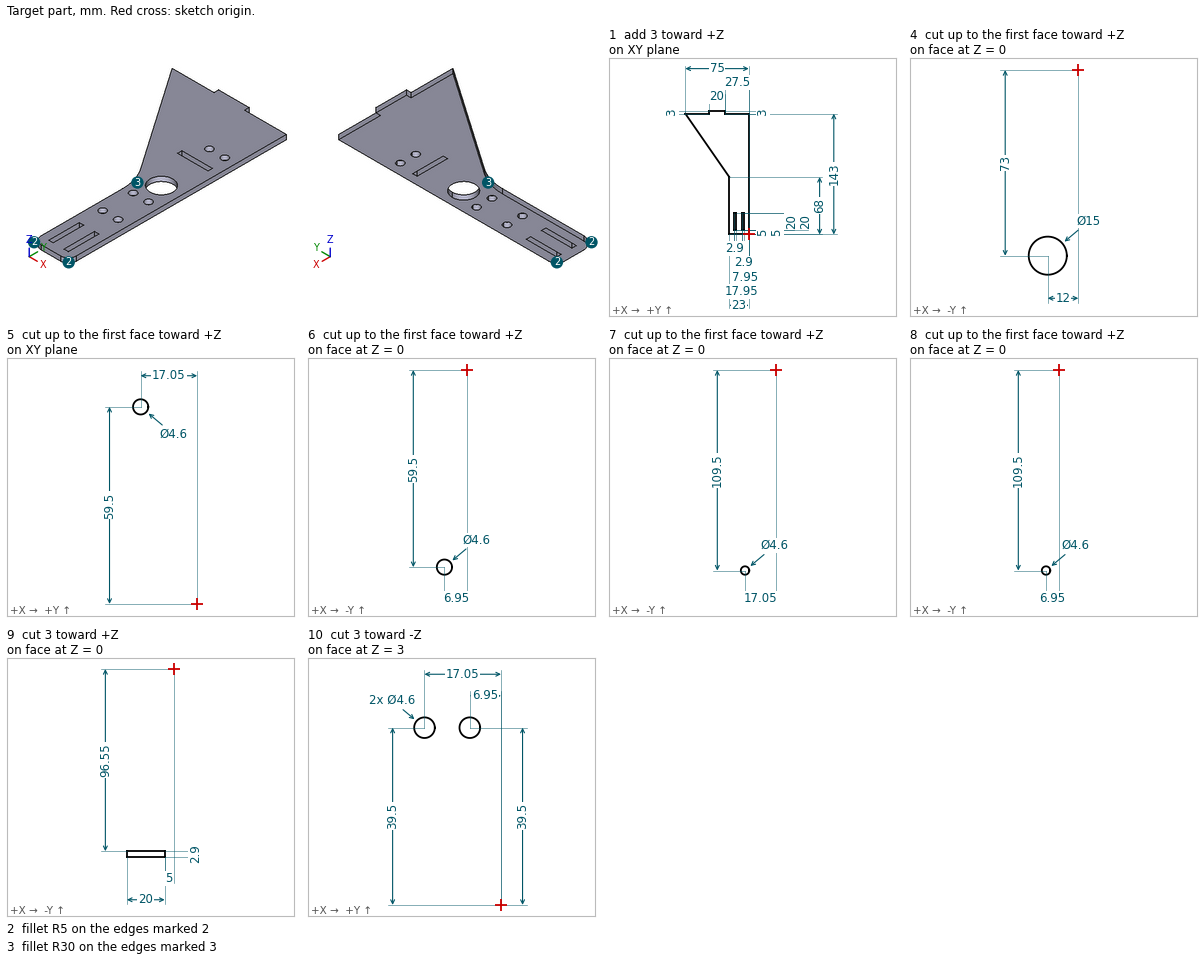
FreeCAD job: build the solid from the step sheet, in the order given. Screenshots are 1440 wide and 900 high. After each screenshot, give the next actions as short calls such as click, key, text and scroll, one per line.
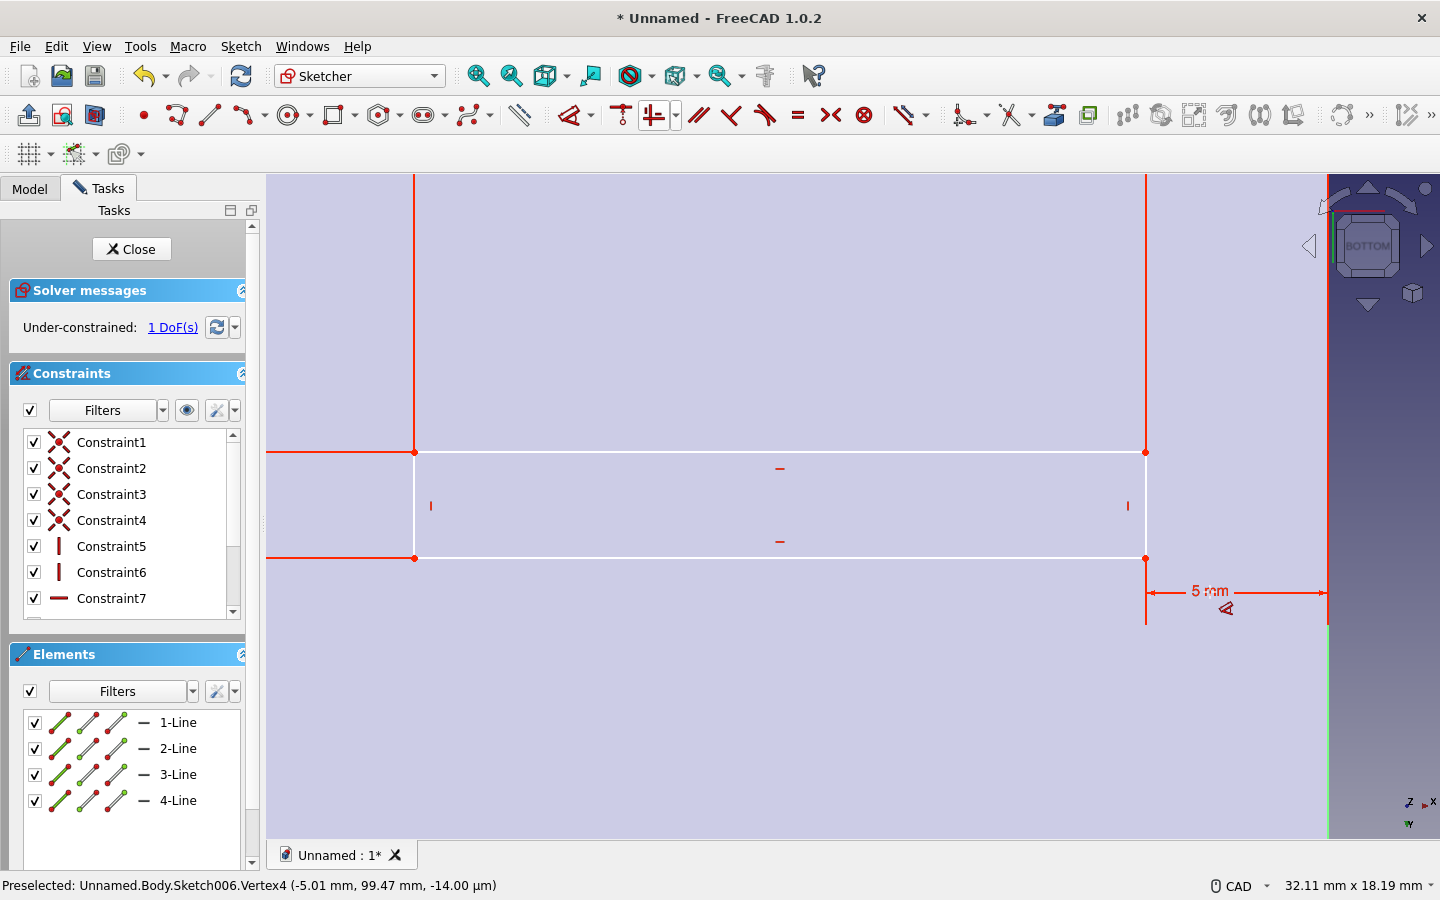
click(414, 452)
click(380, 327)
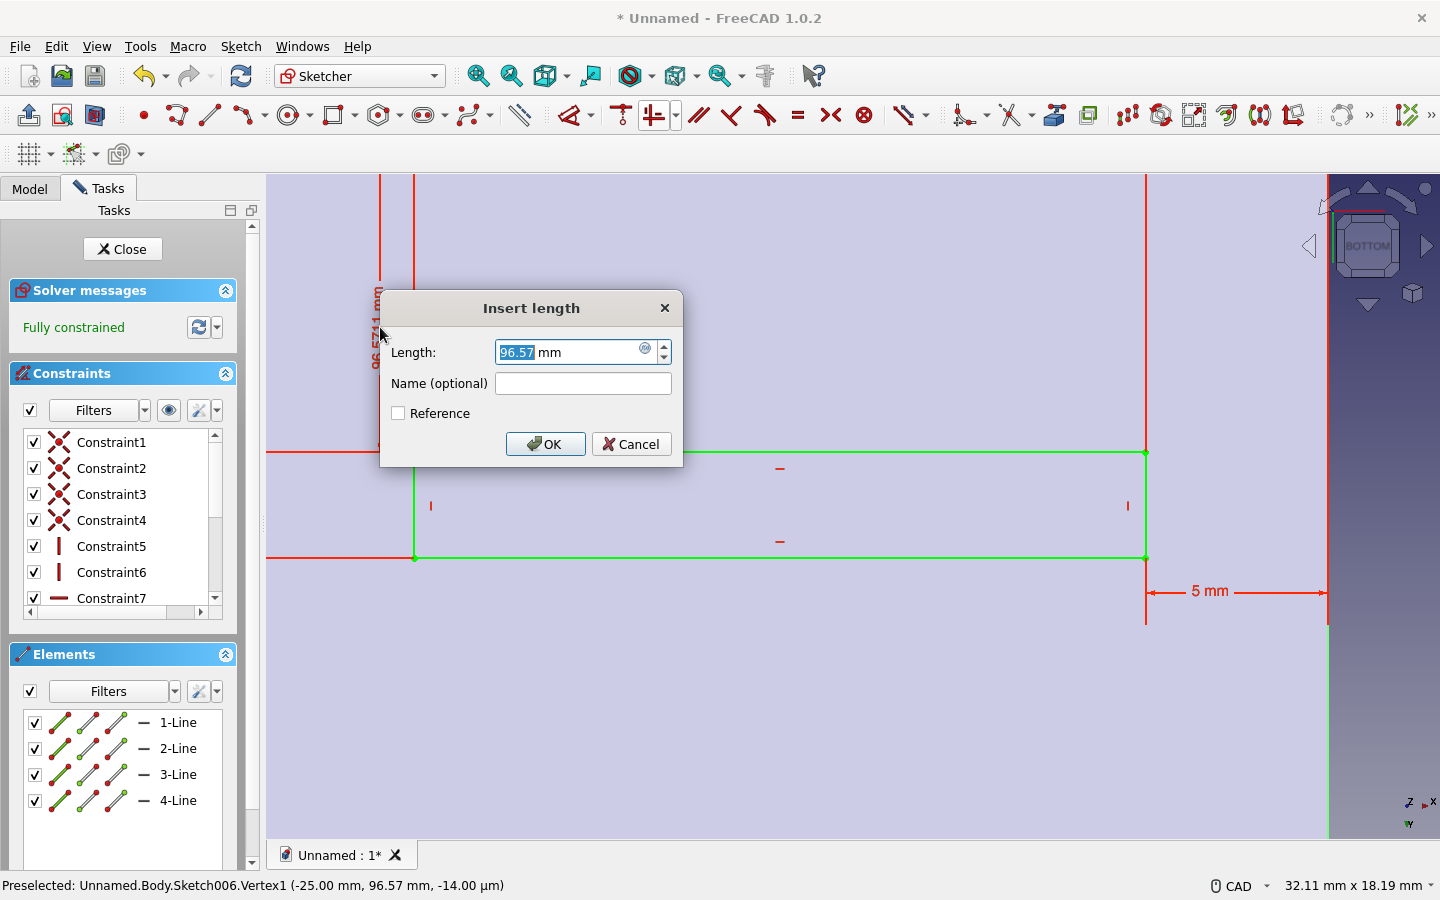
text(96.55)
key(Return)
key(Escape)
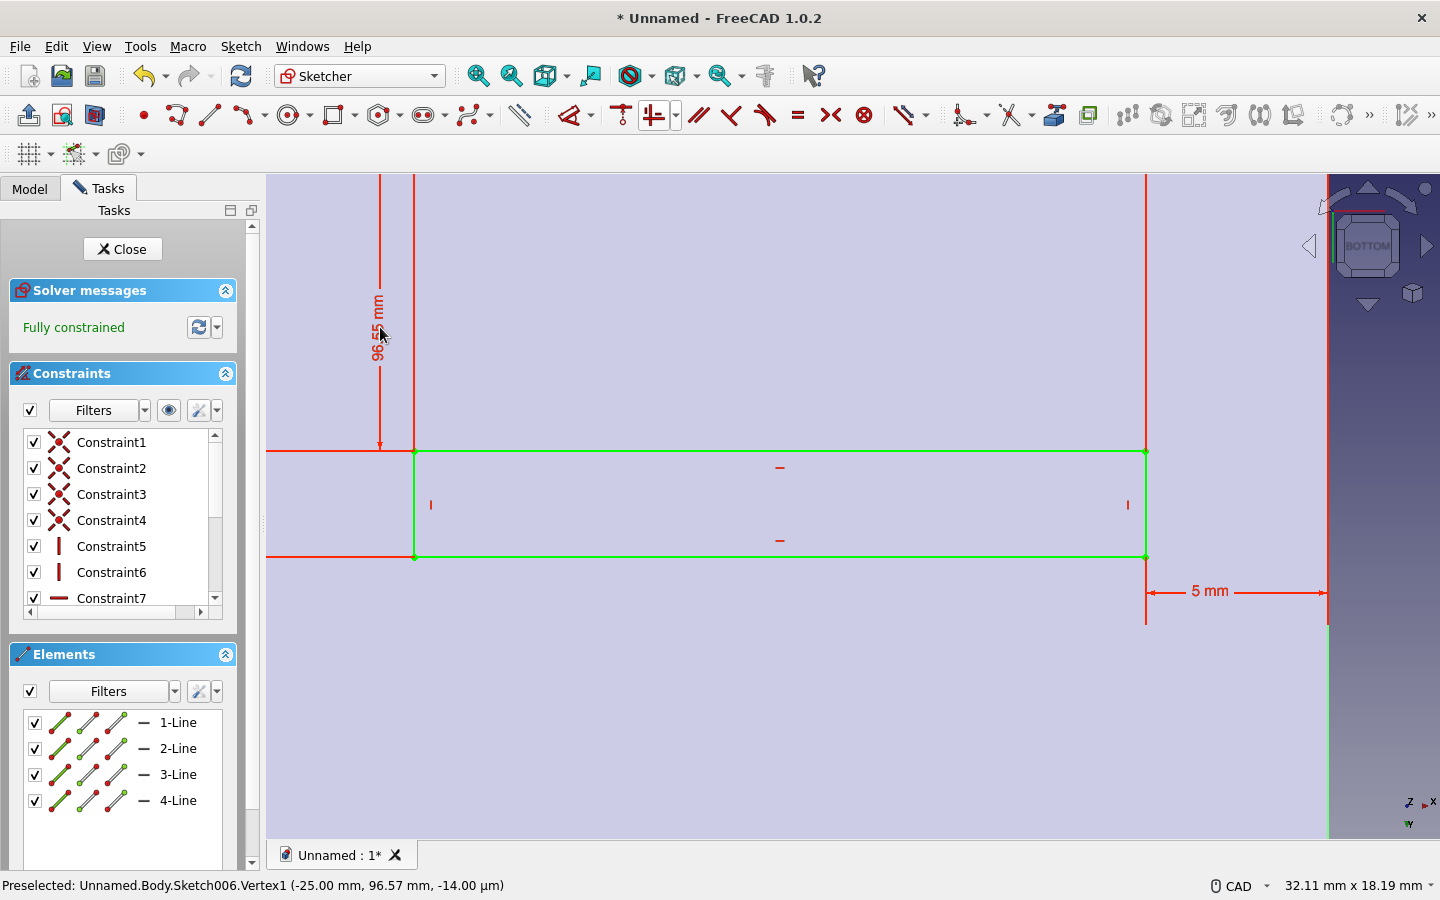
click(123, 249)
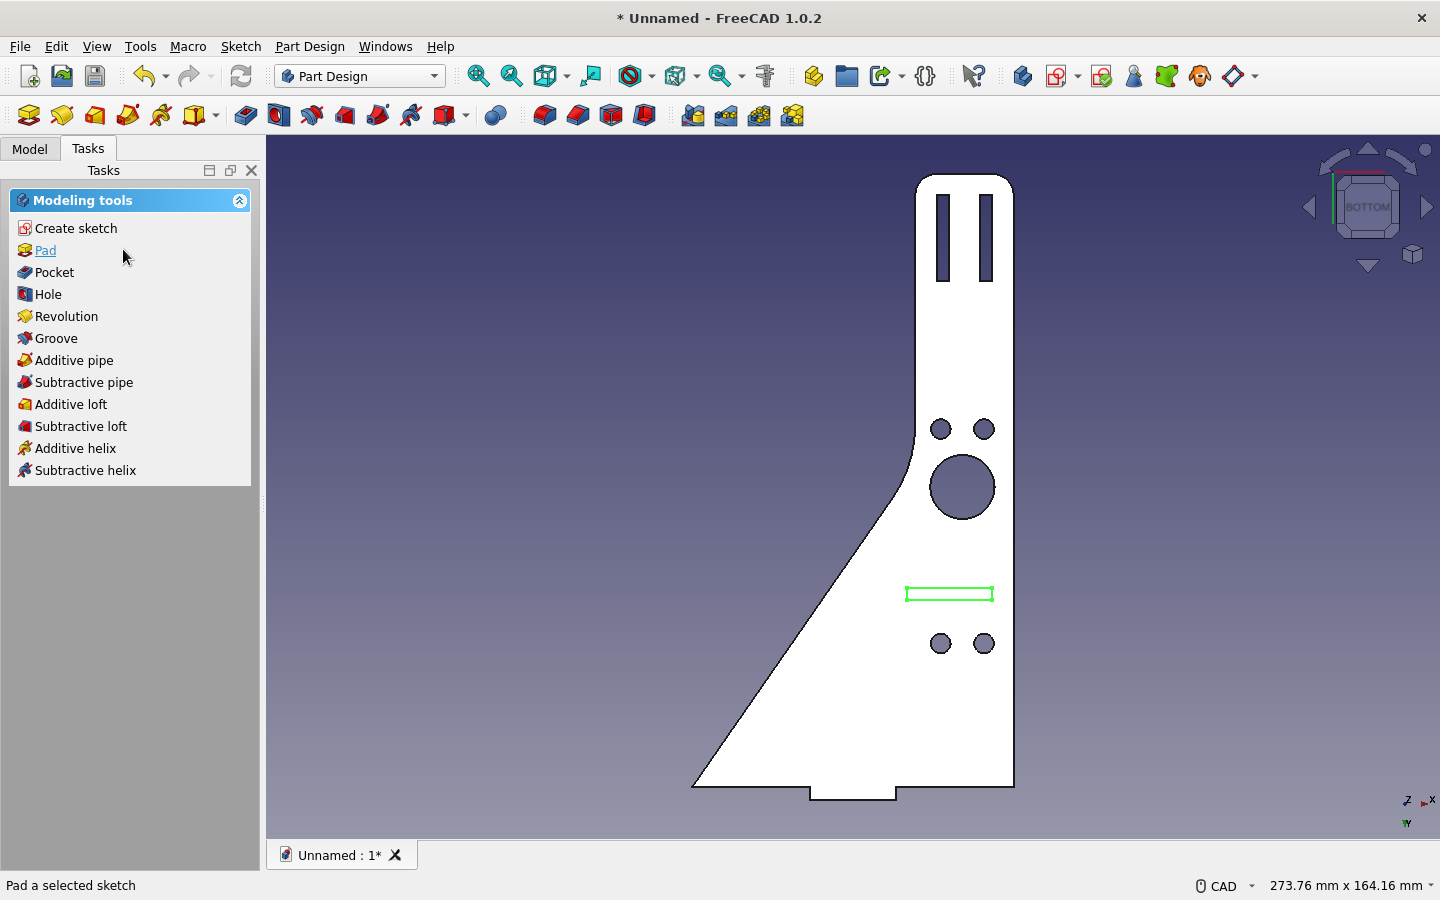
click(246, 116)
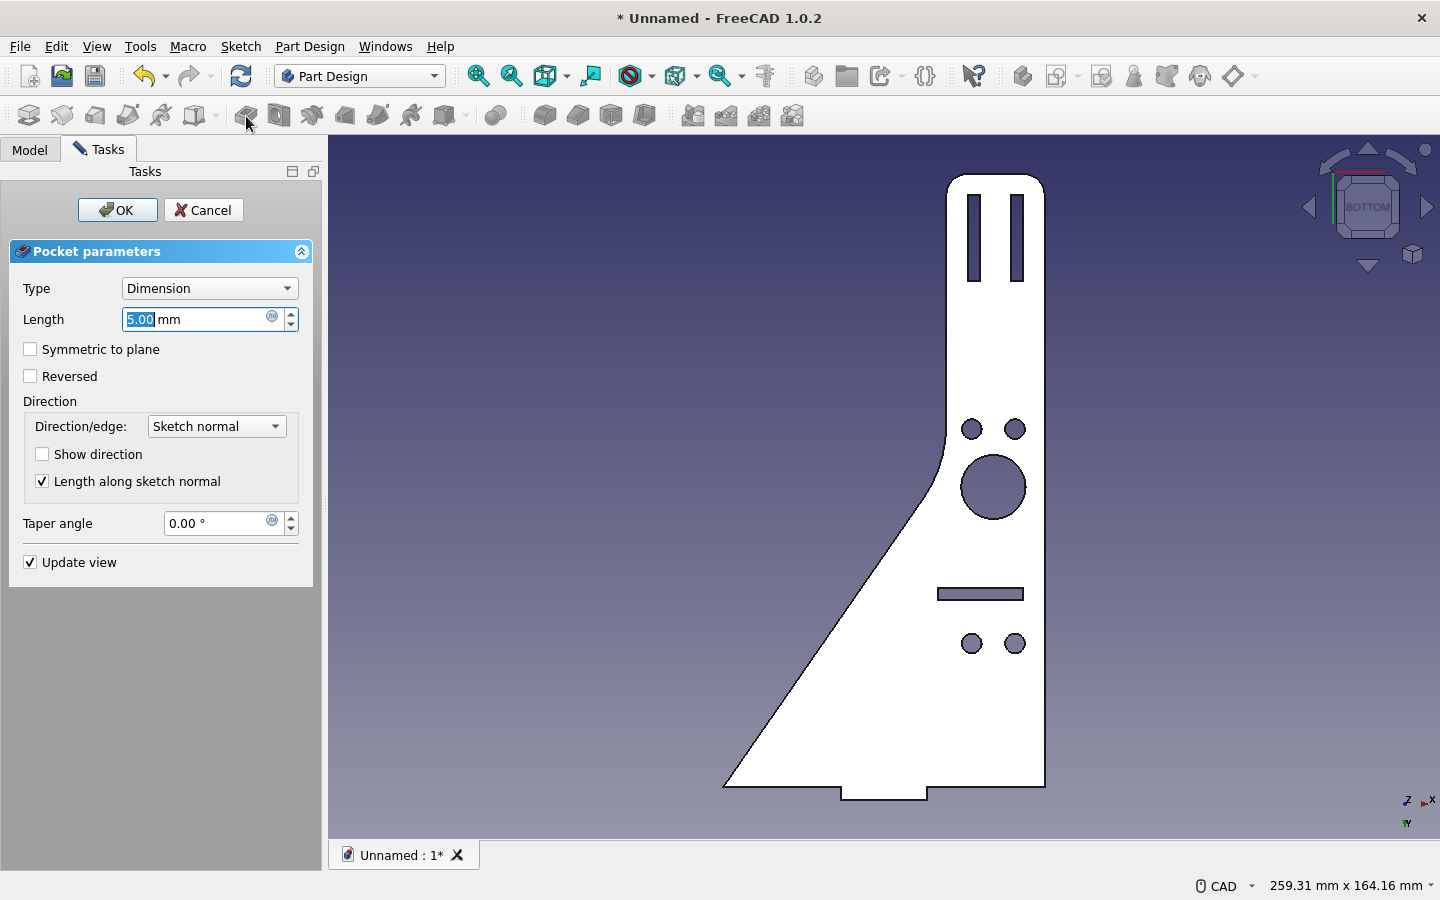
text(3)
key(Tab)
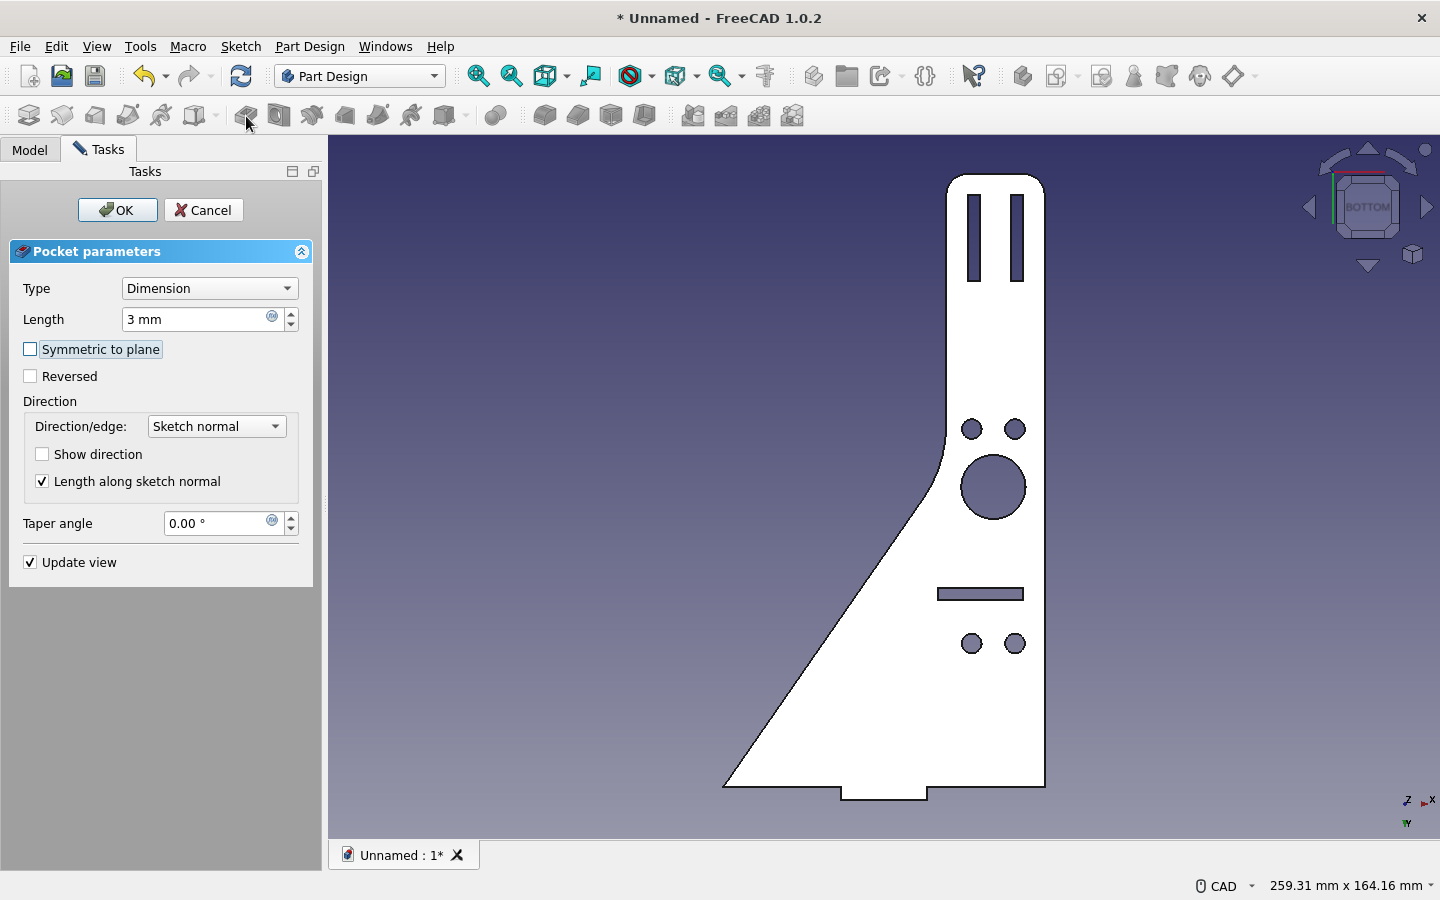
click(118, 210)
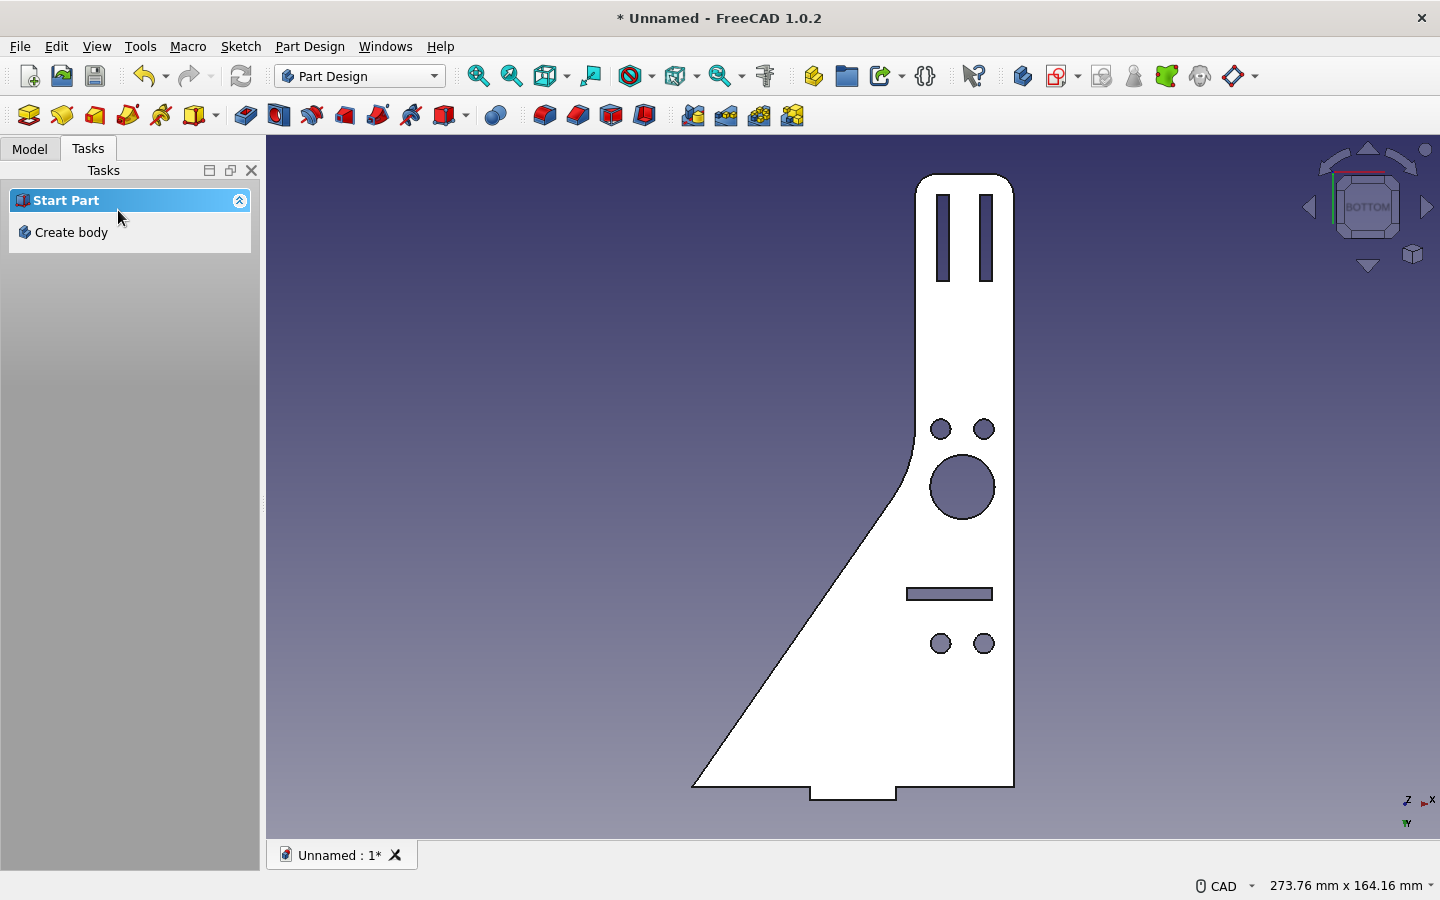
key(0)